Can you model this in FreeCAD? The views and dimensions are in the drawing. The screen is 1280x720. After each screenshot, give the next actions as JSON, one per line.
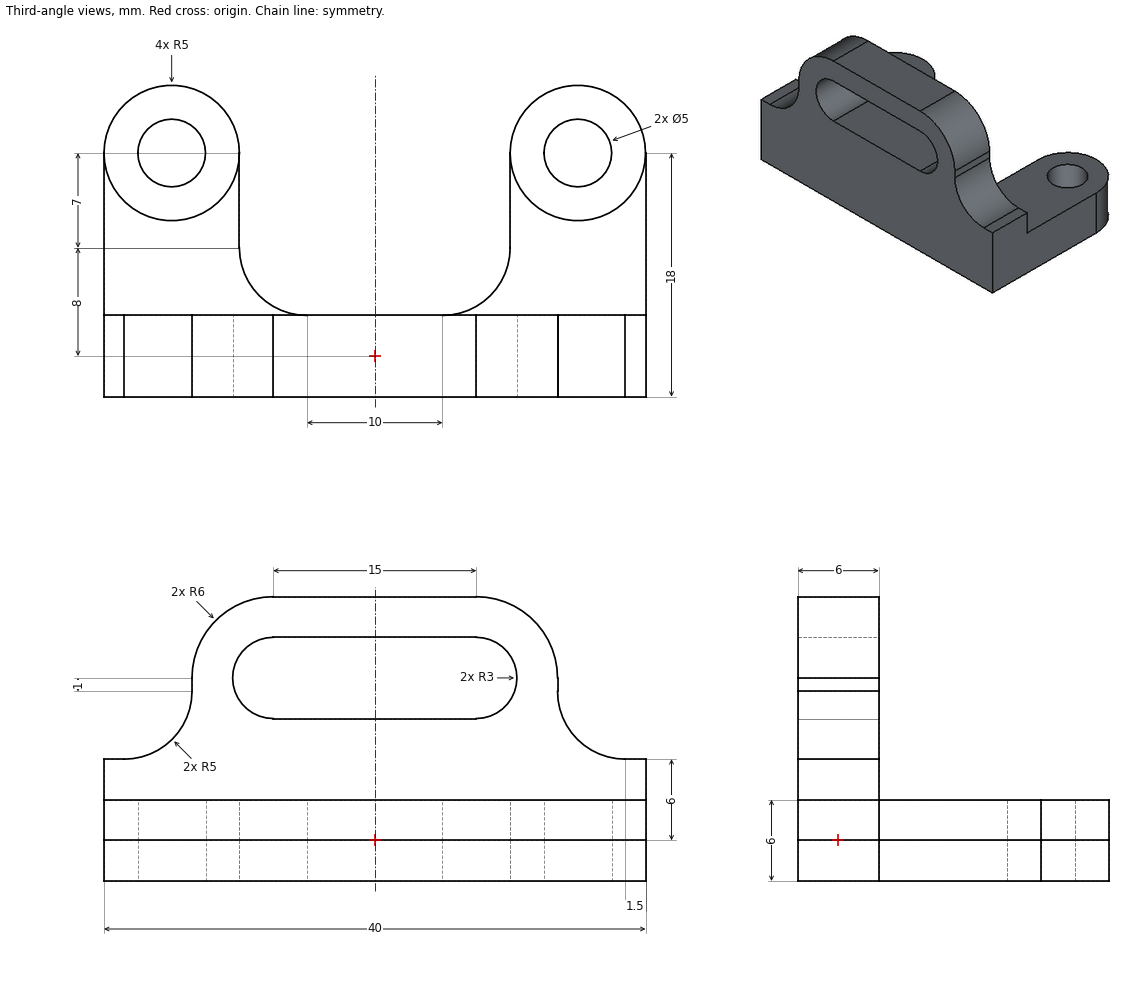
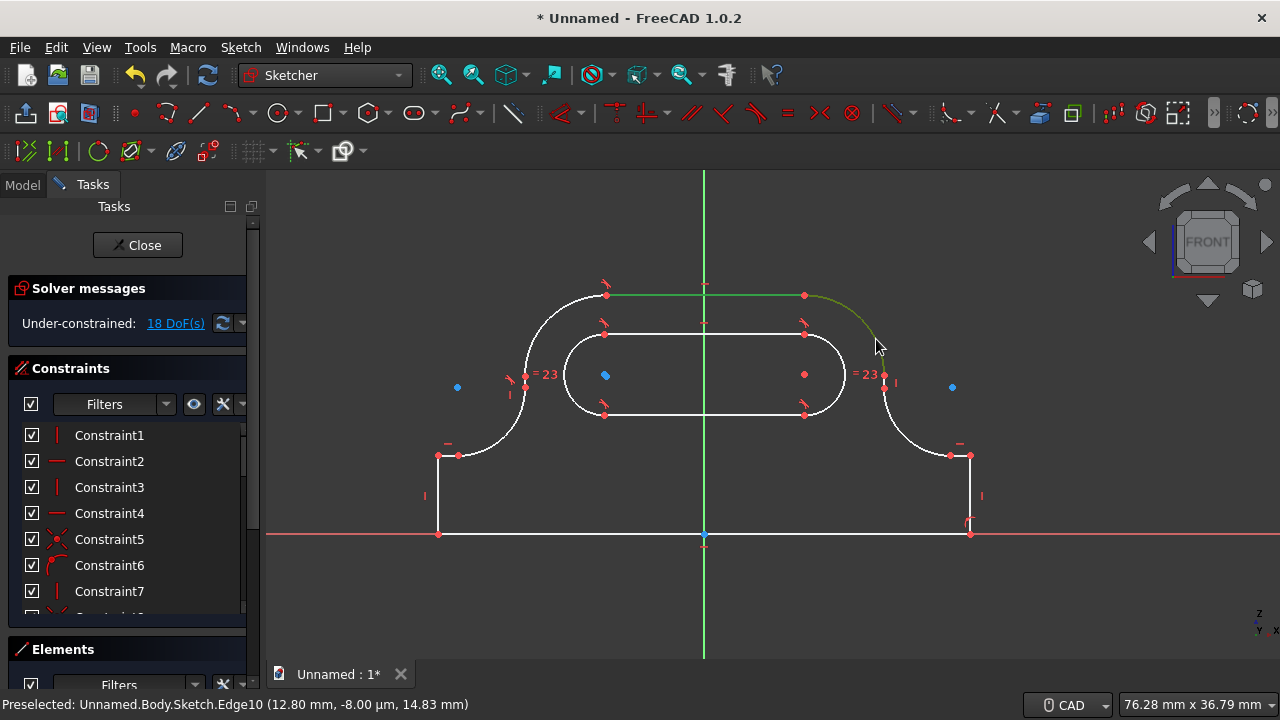
{"action": "key", "text": "t"}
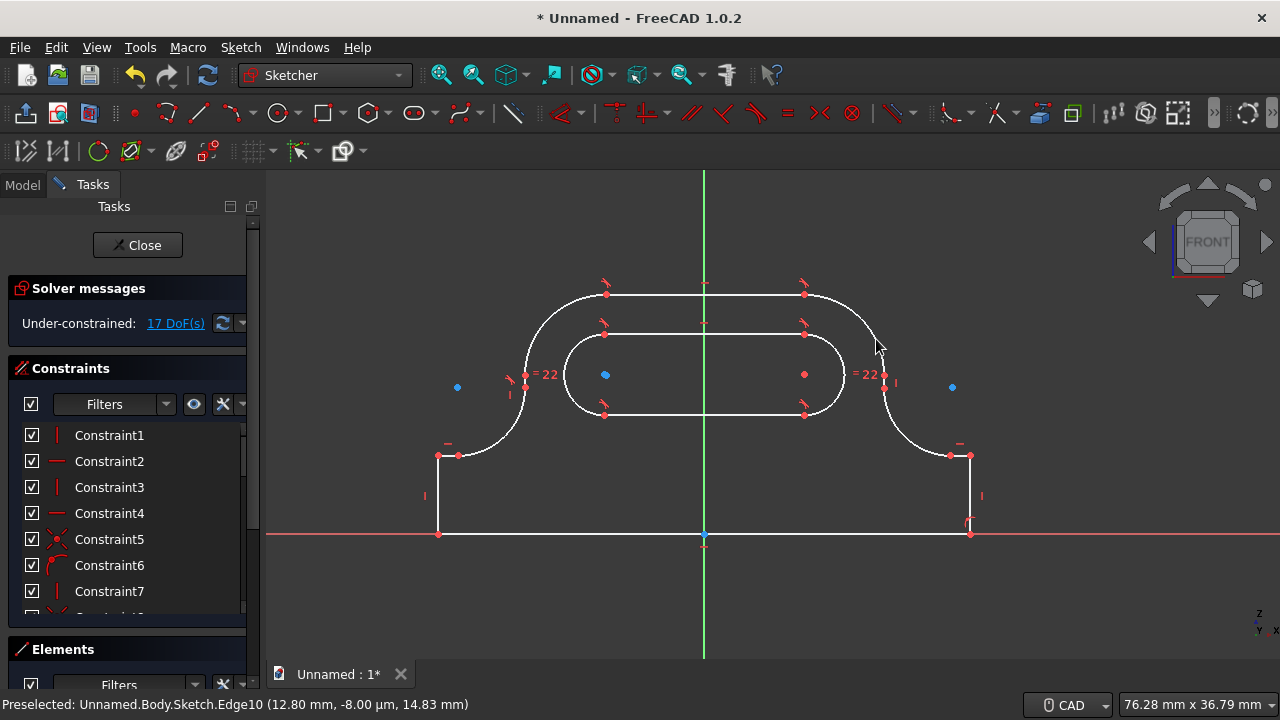
{"action": "scroll", "coordinate": [884, 382], "scroll_direction": "up", "scroll_amount": 4}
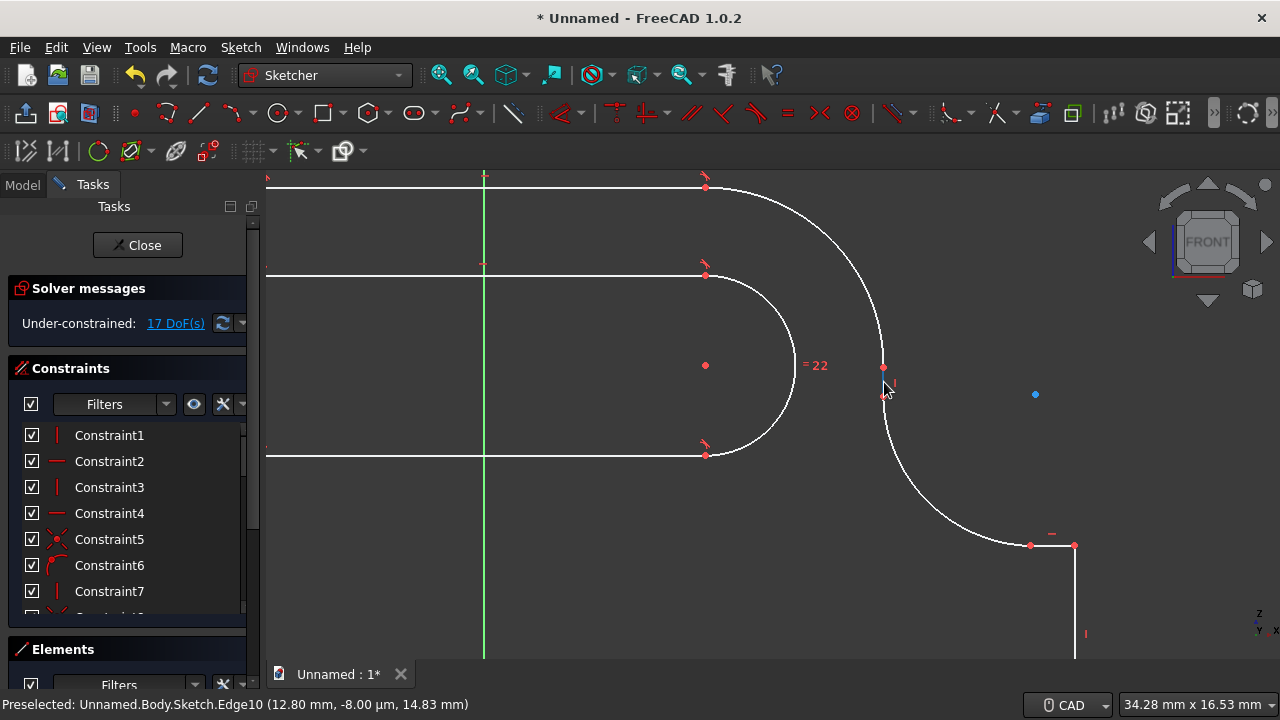
{"action": "left_click", "coordinate": [883, 382]}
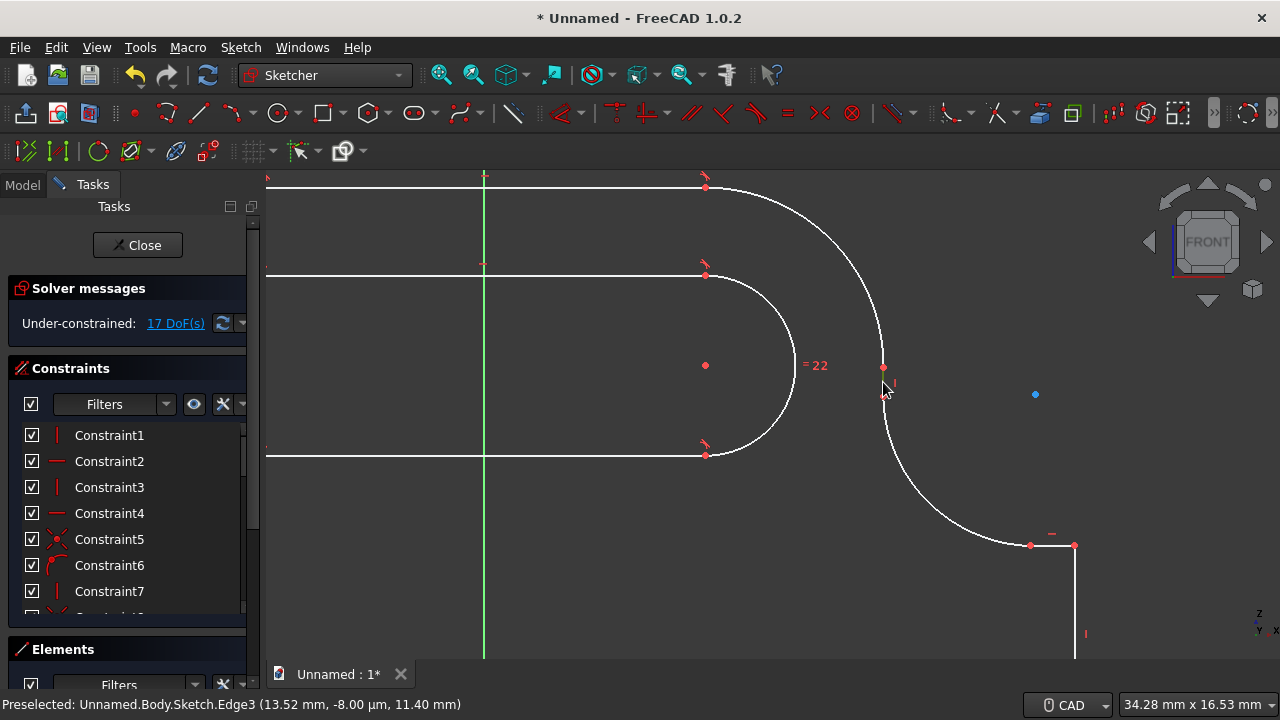
{"action": "left_click", "coordinate": [865, 286]}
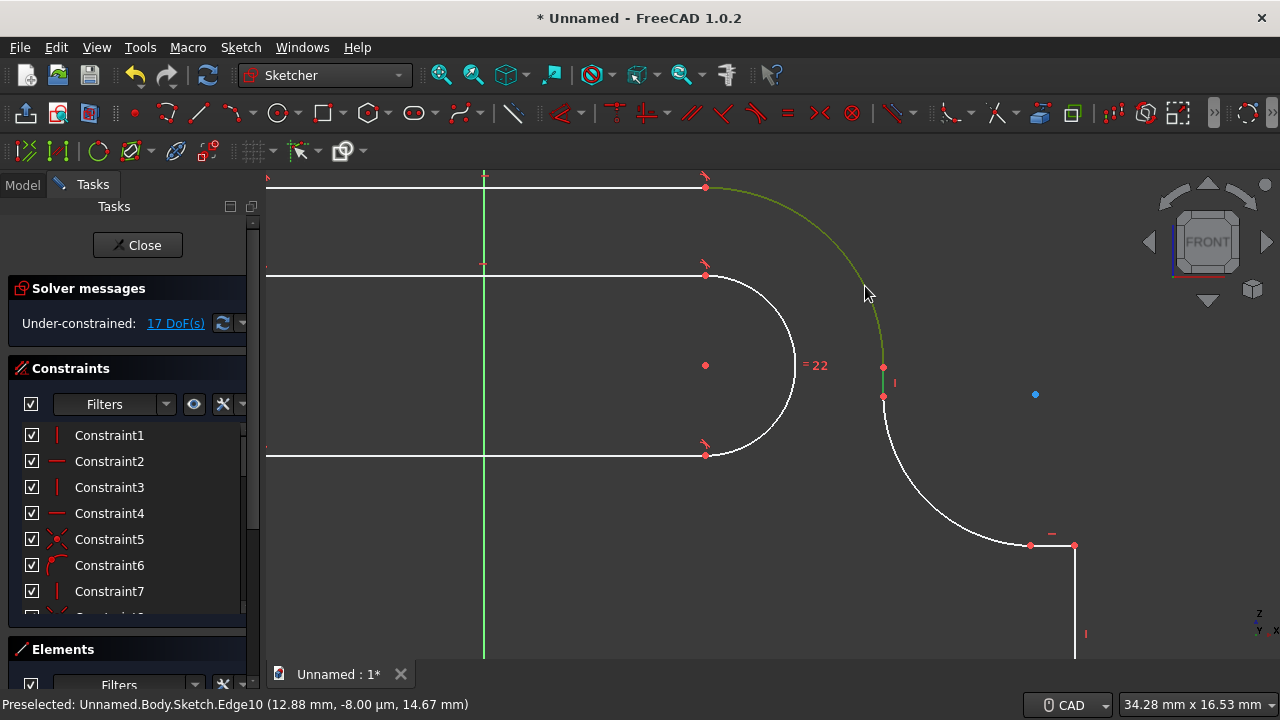
{"action": "key", "text": "t"}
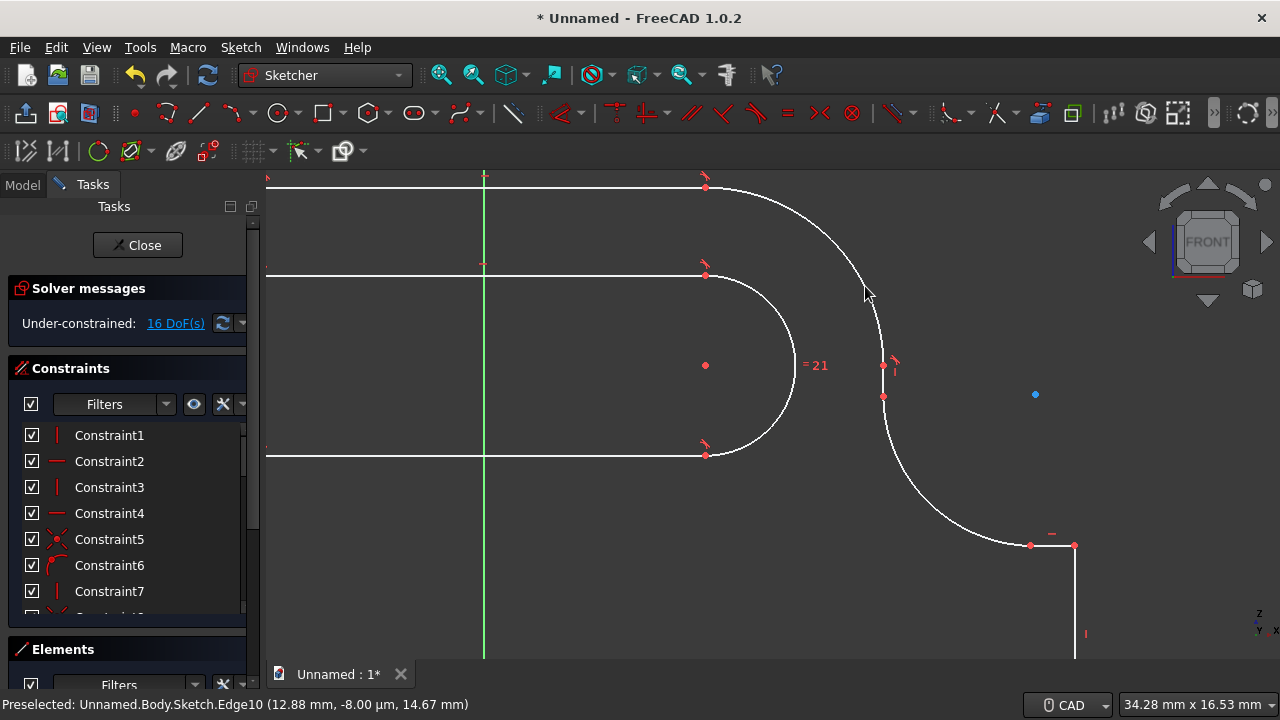
{"action": "scroll", "coordinate": [883, 375], "scroll_direction": "up", "scroll_amount": 2}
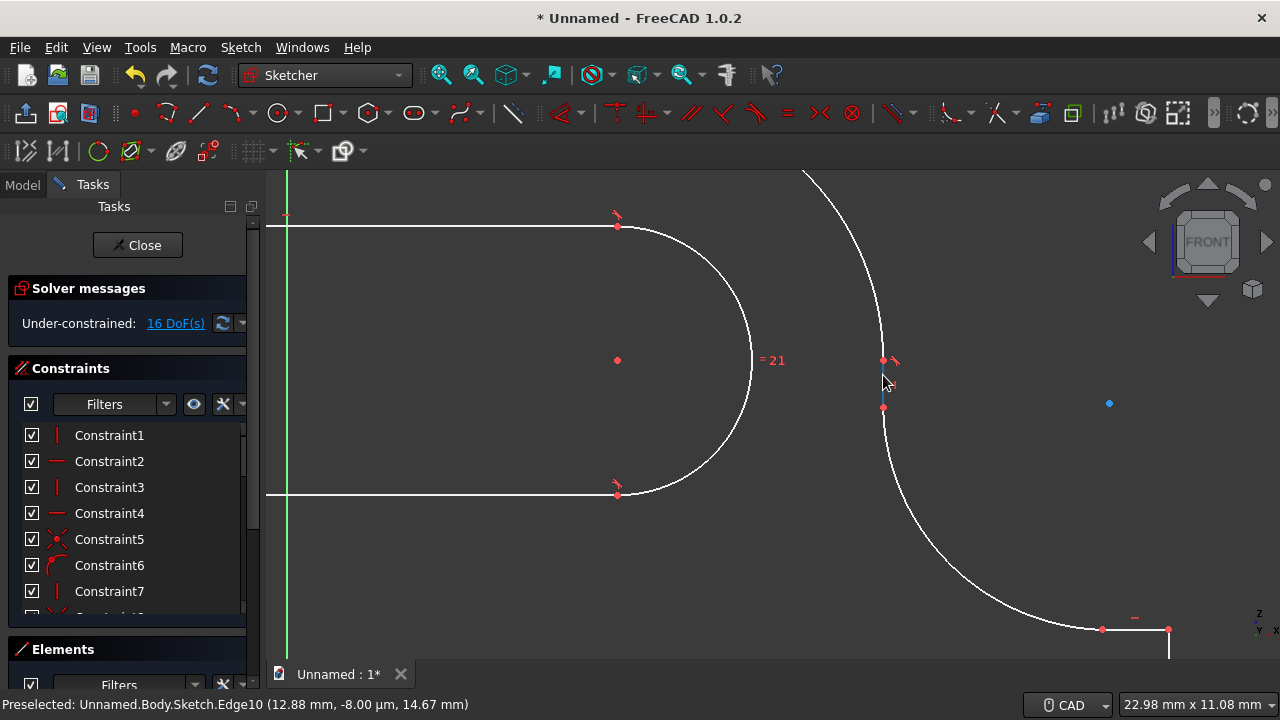
{"action": "left_click", "coordinate": [883, 375]}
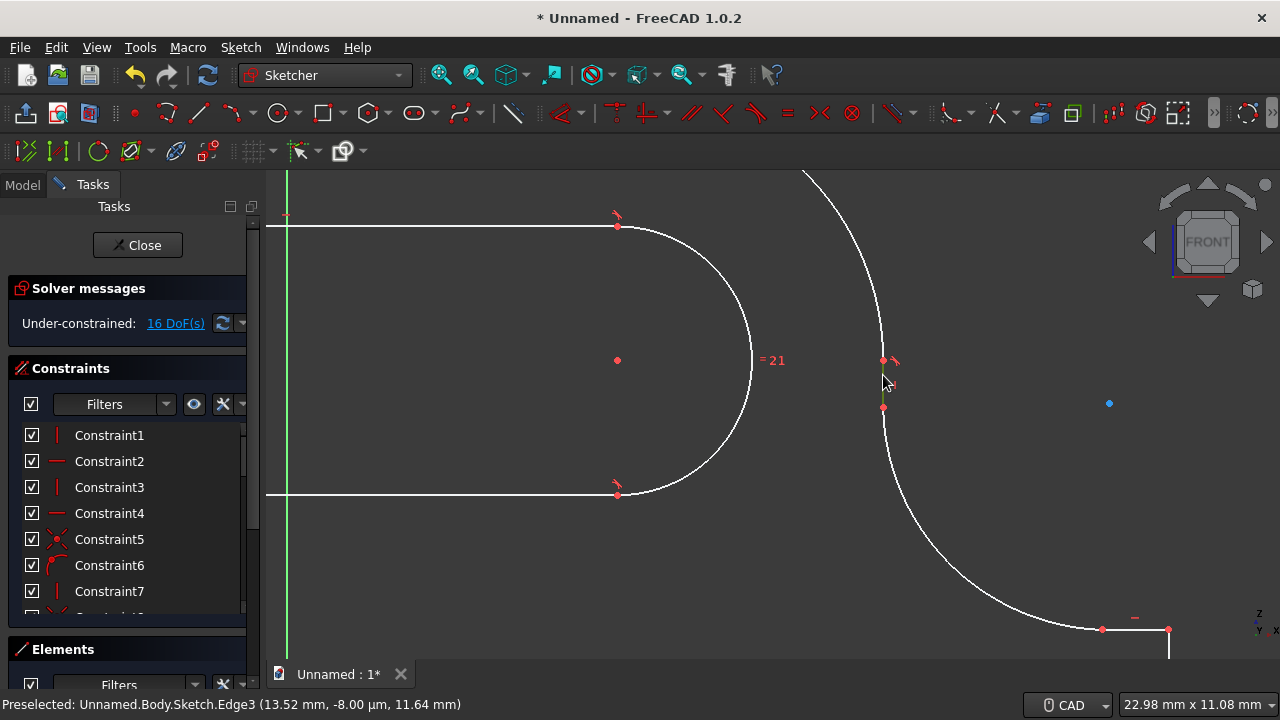
{"action": "left_click", "coordinate": [908, 507]}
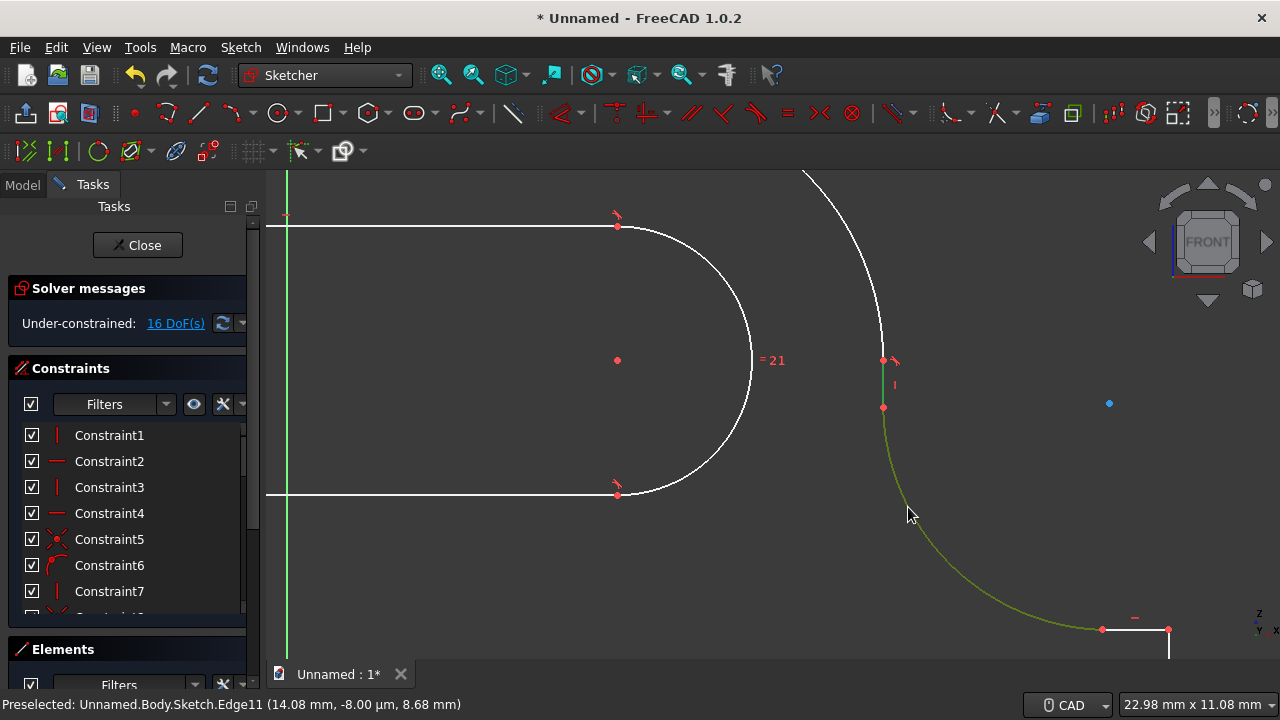
{"action": "left_click", "coordinate": [756, 114]}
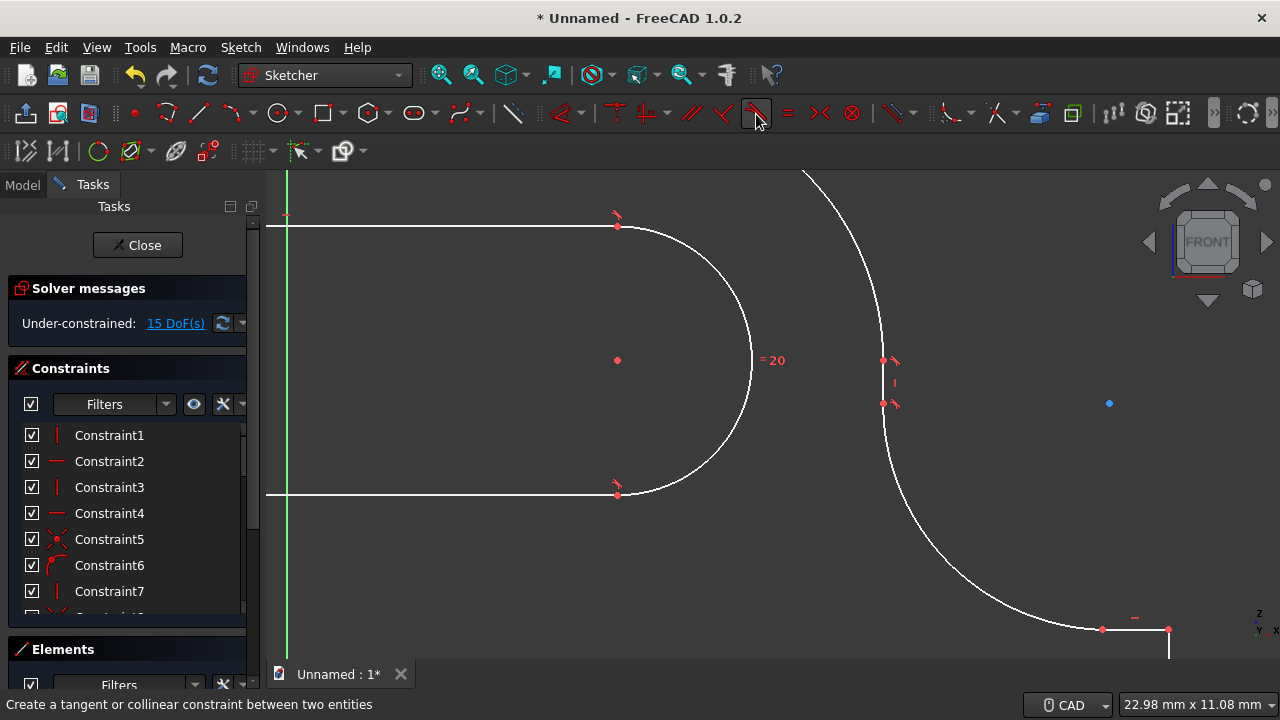
{"action": "scroll", "coordinate": [885, 381], "scroll_direction": "down", "scroll_amount": 6}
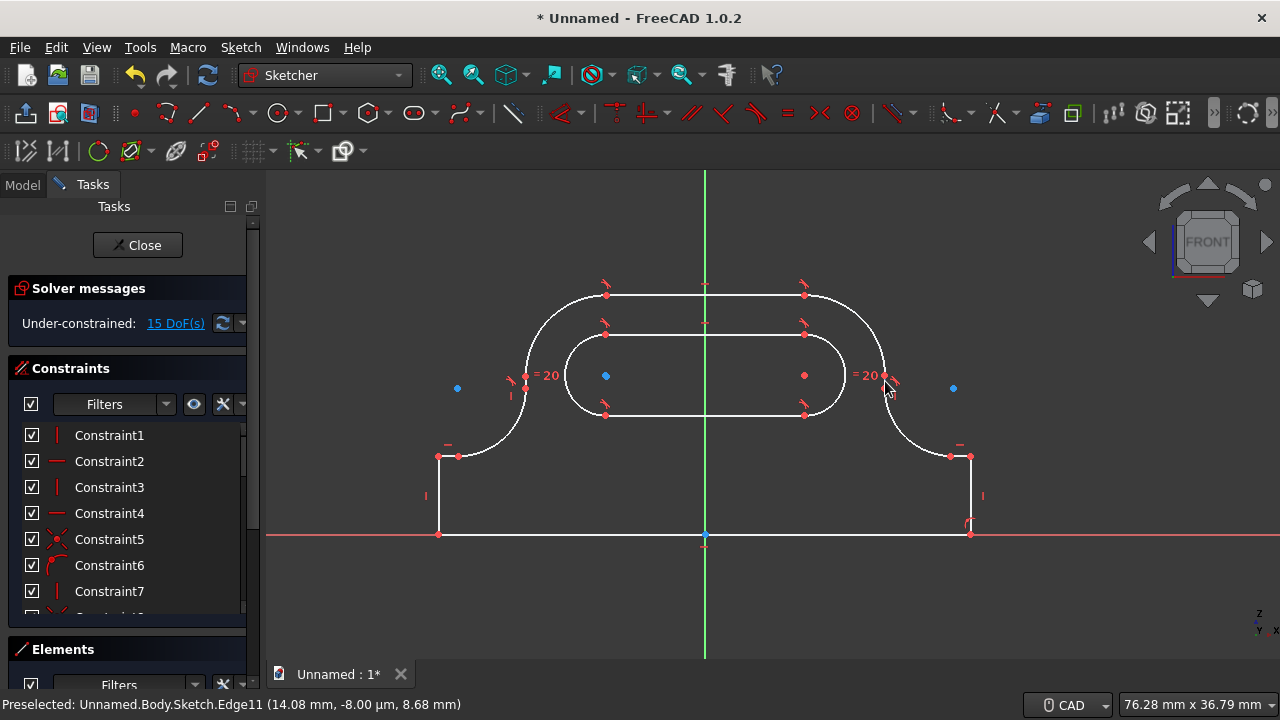
{"action": "scroll", "coordinate": [957, 456], "scroll_direction": "up", "scroll_amount": 5}